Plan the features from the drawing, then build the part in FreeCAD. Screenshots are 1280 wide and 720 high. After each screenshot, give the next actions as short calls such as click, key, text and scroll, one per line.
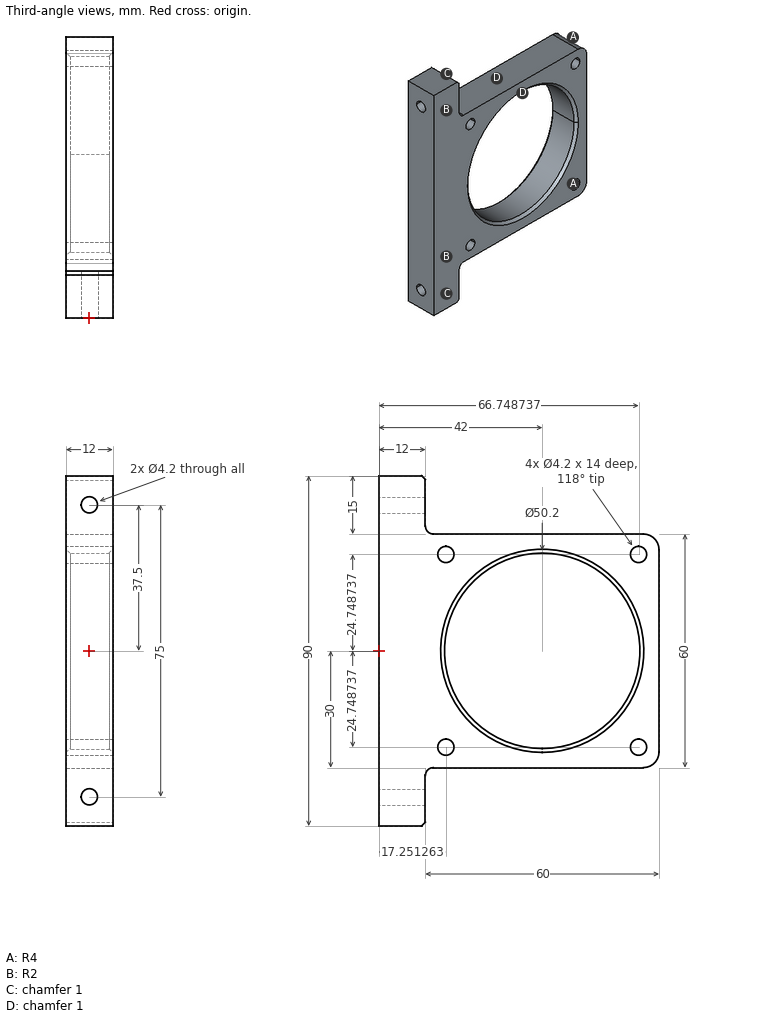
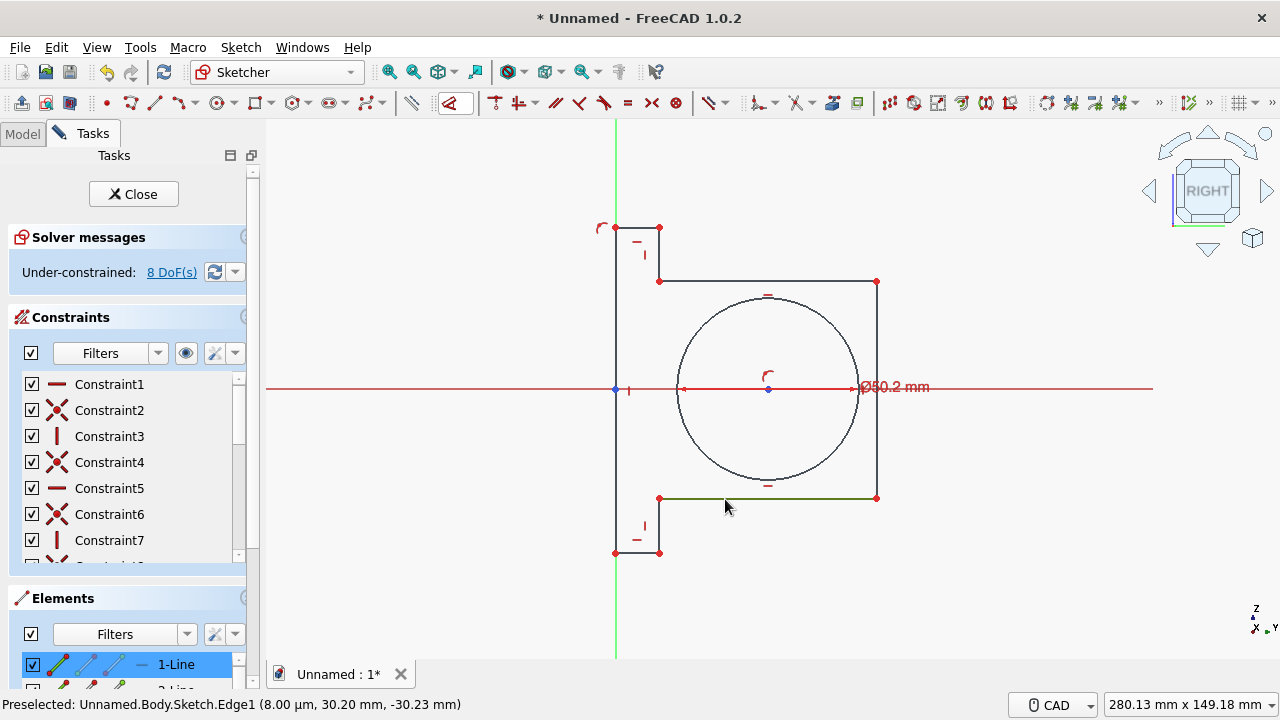
click(468, 104)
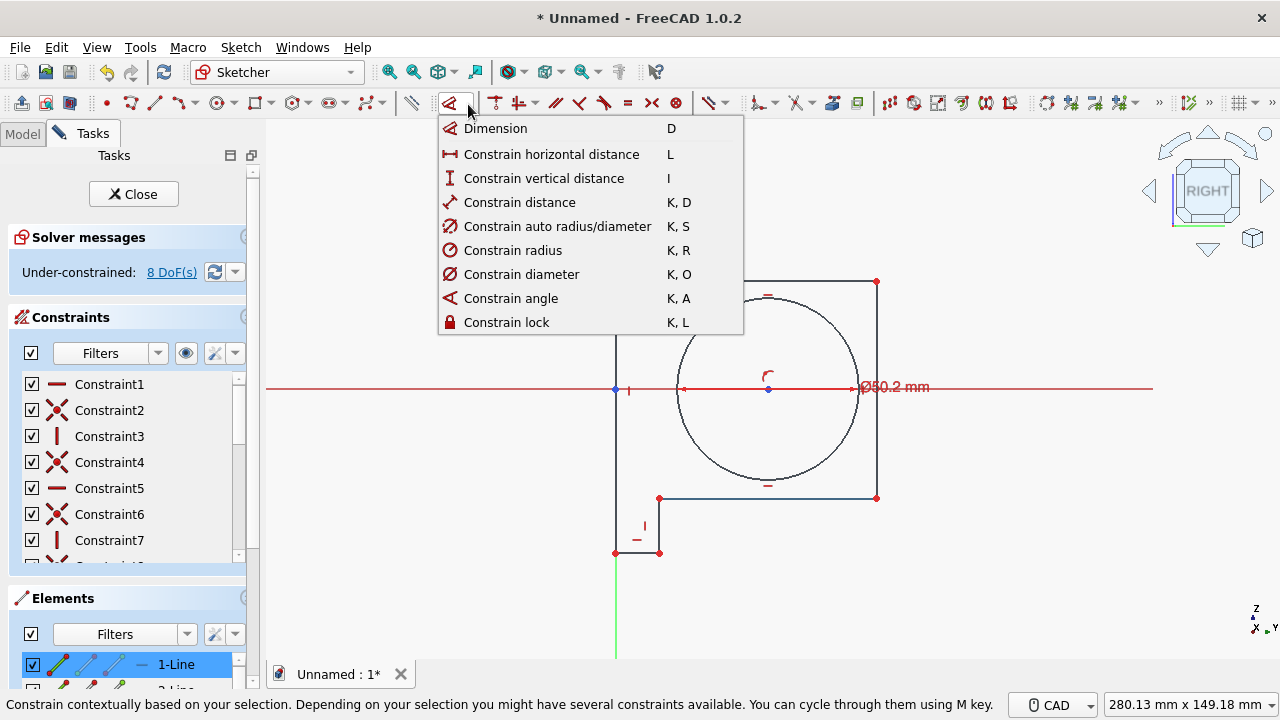
click(591, 154)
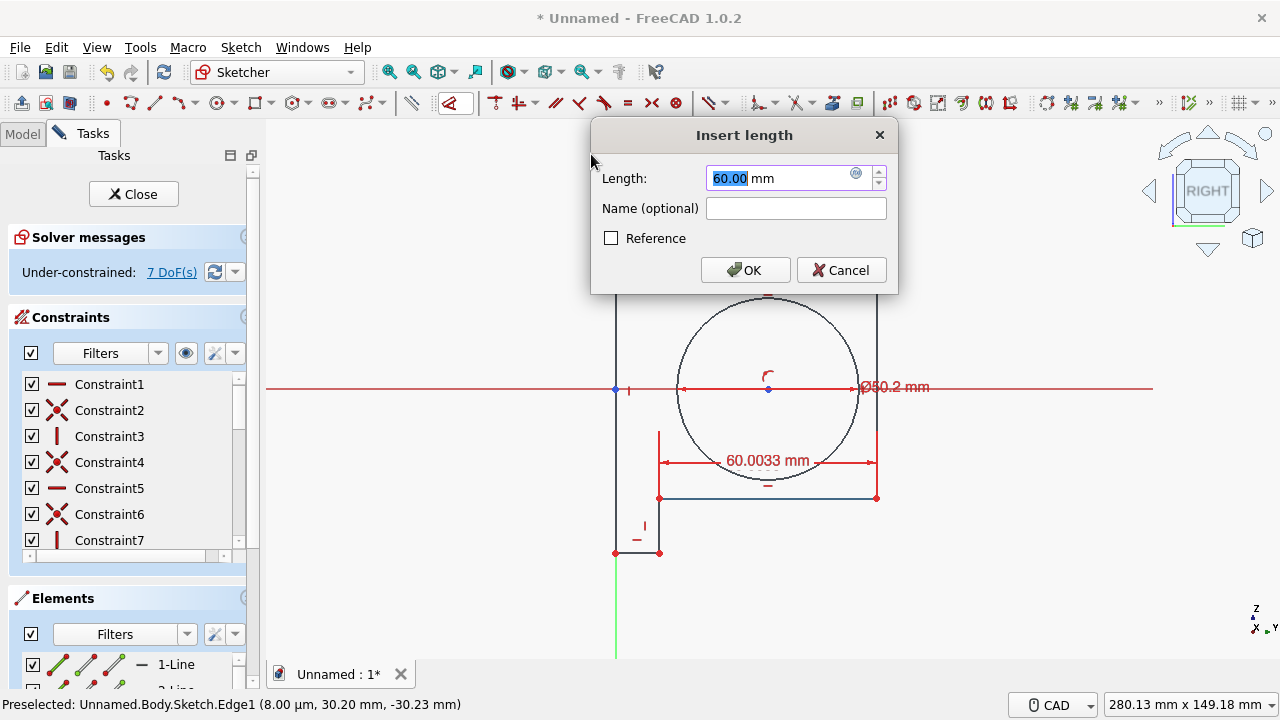
text(60)
key(Return)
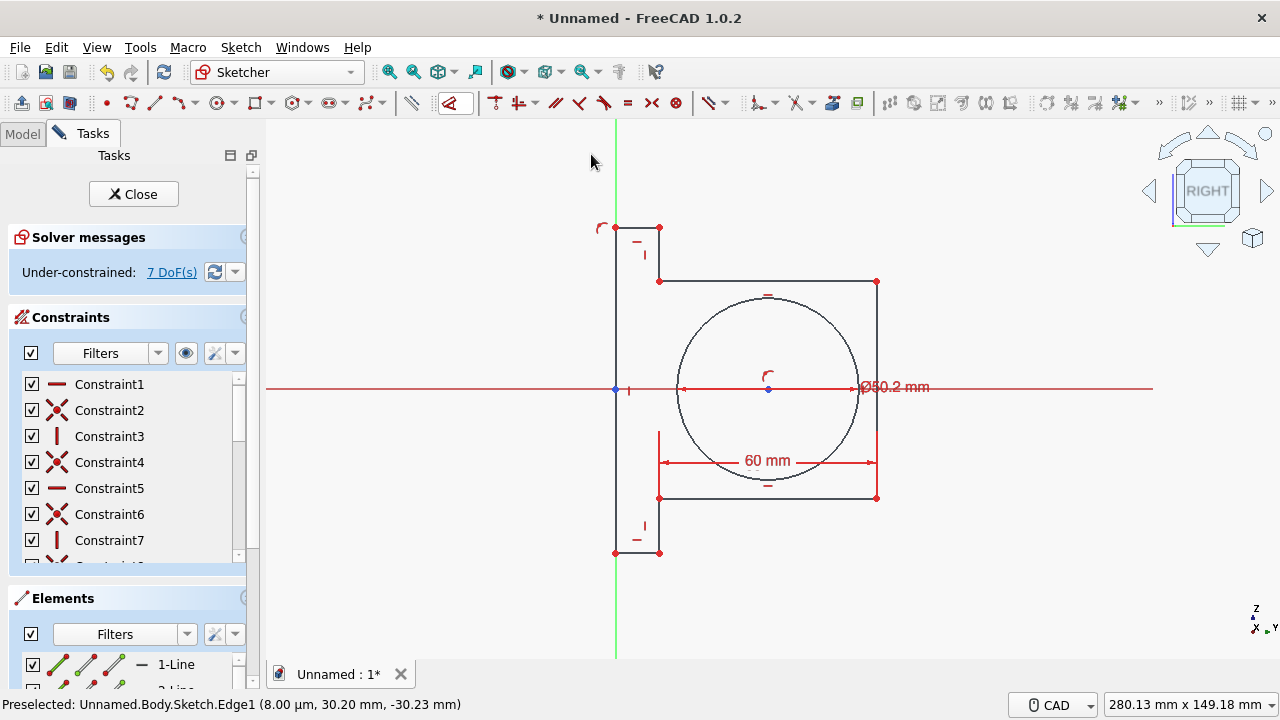
click(877, 433)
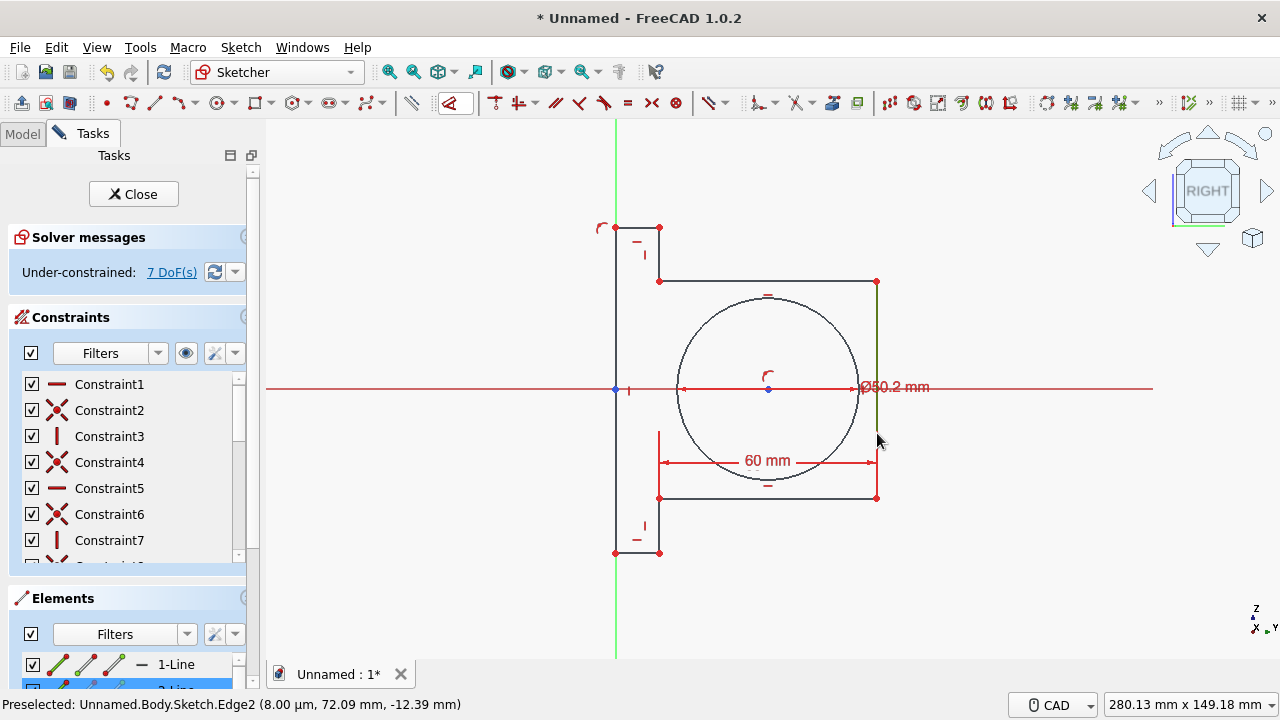
click(468, 104)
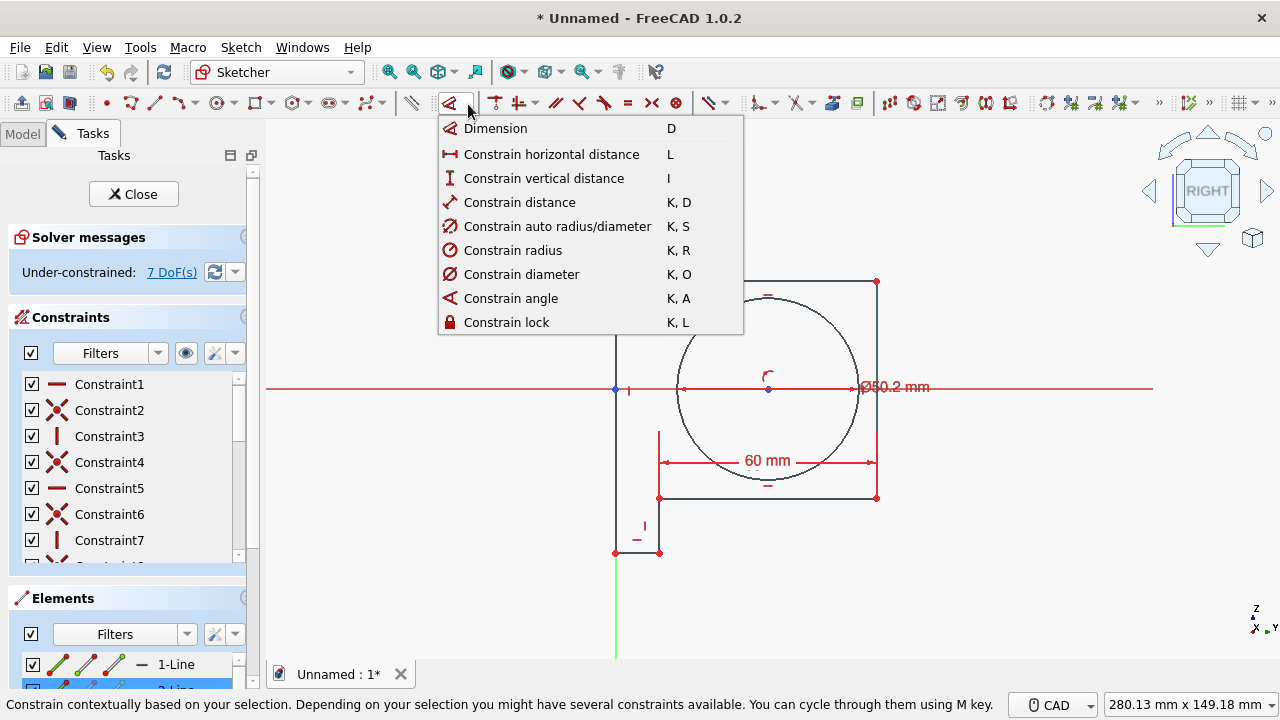
click(591, 178)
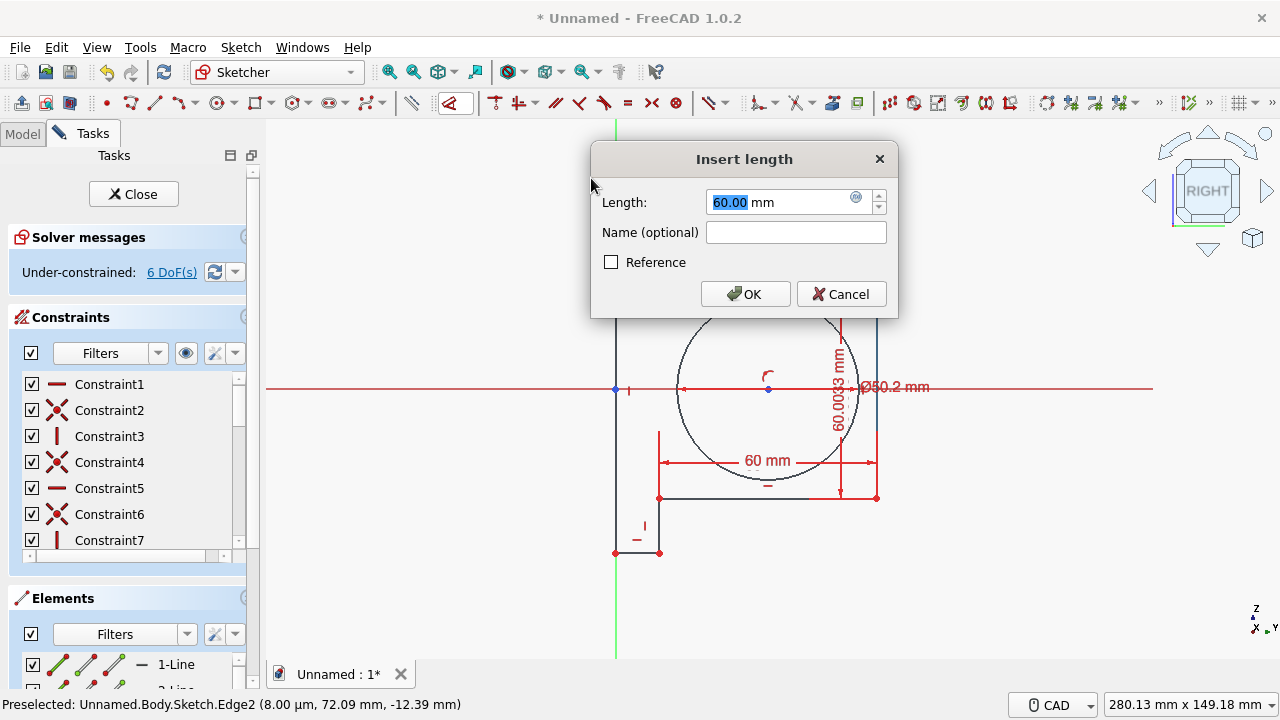
text(60)
key(Return)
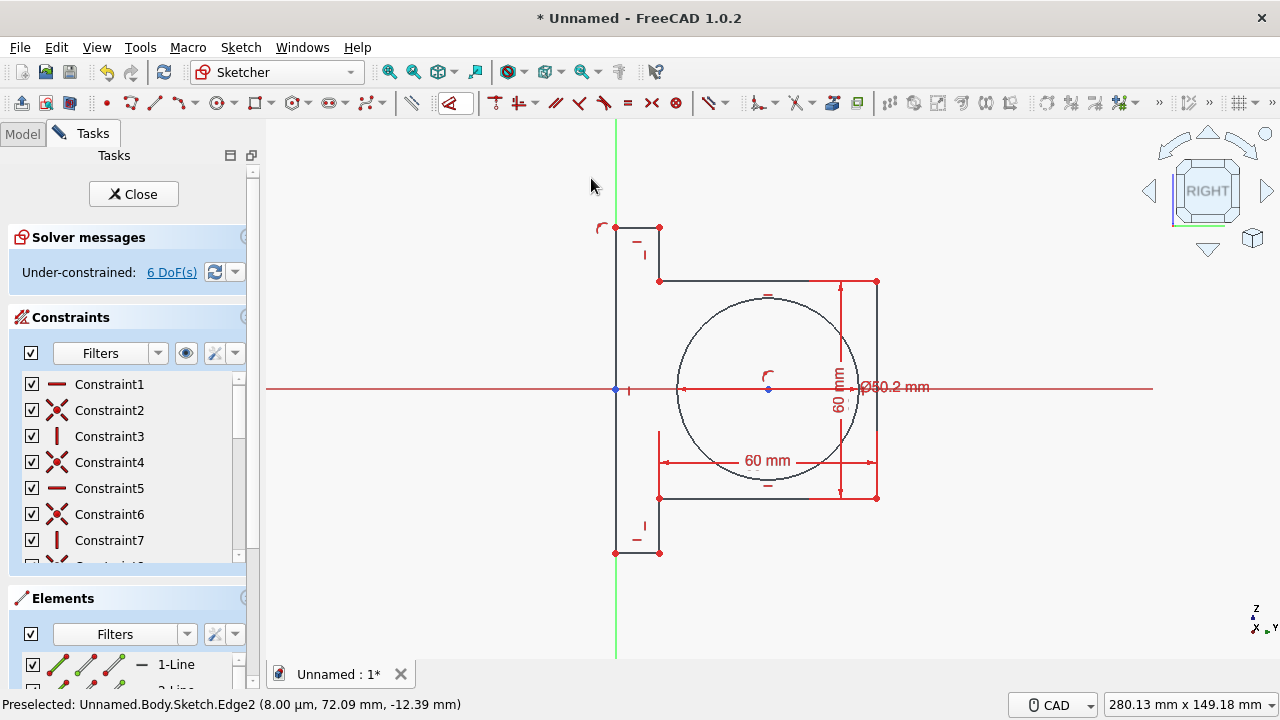
click(811, 281)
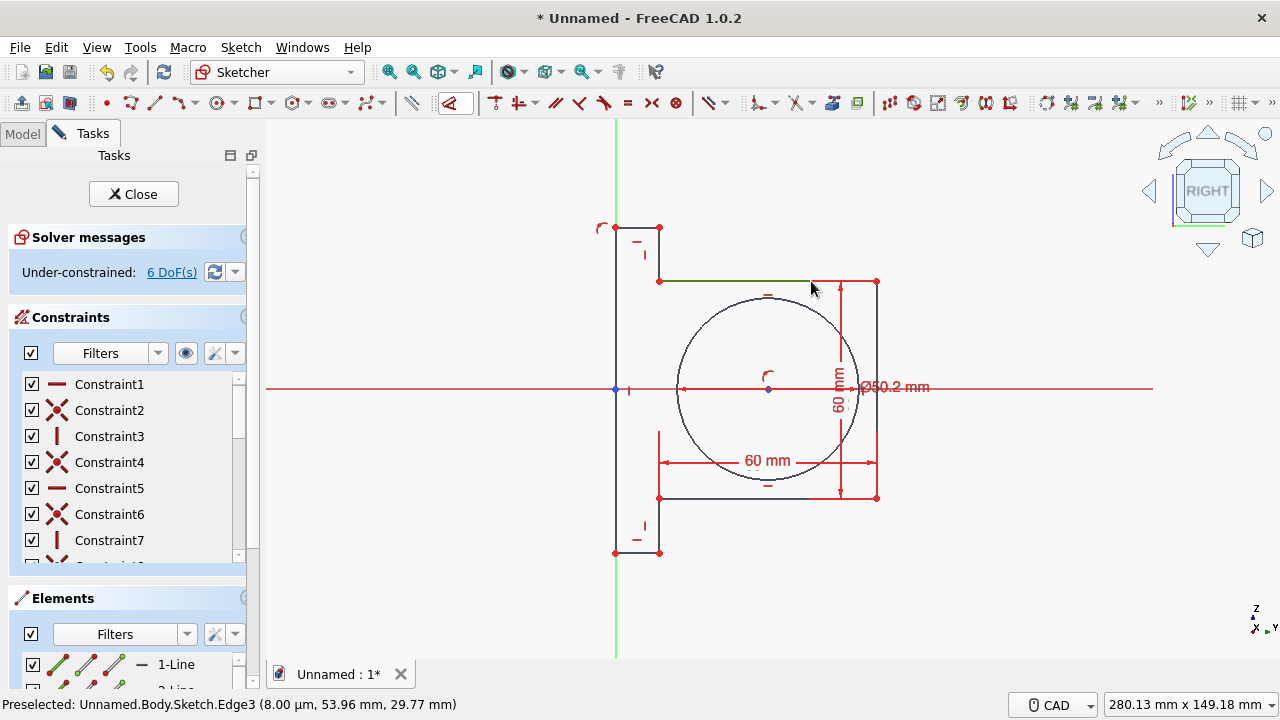
key(l)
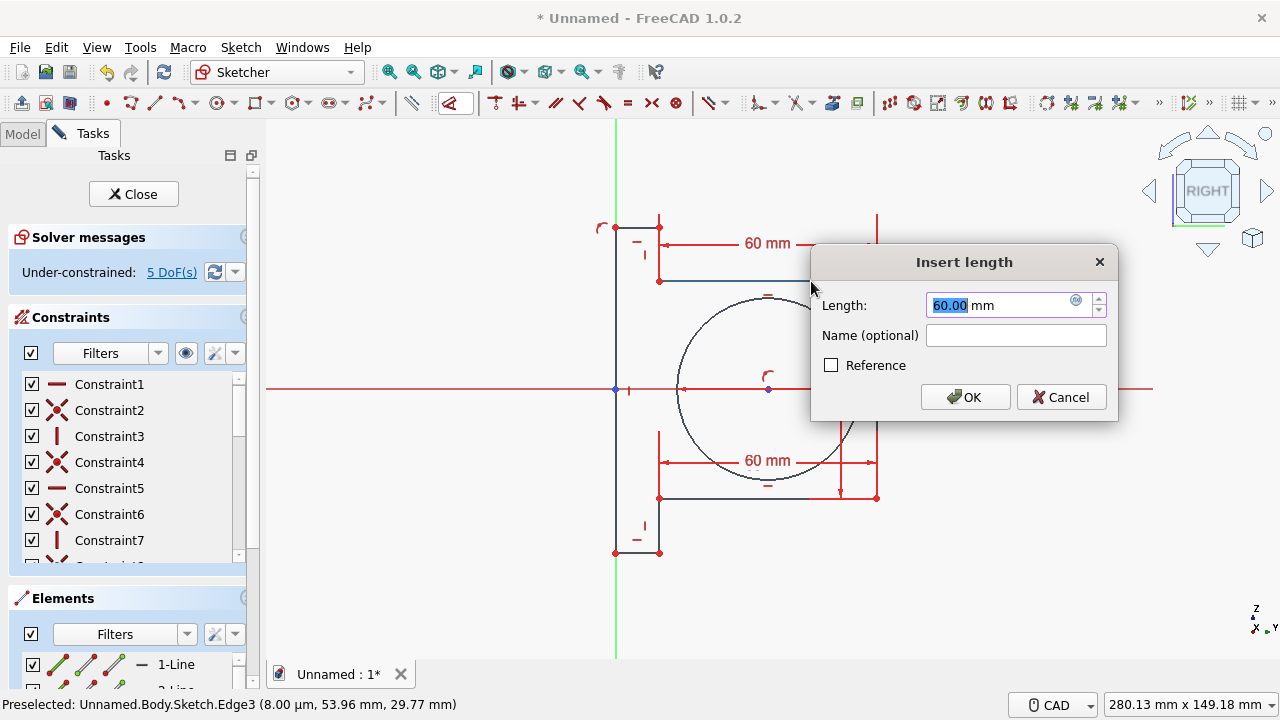
text(60)
key(Return)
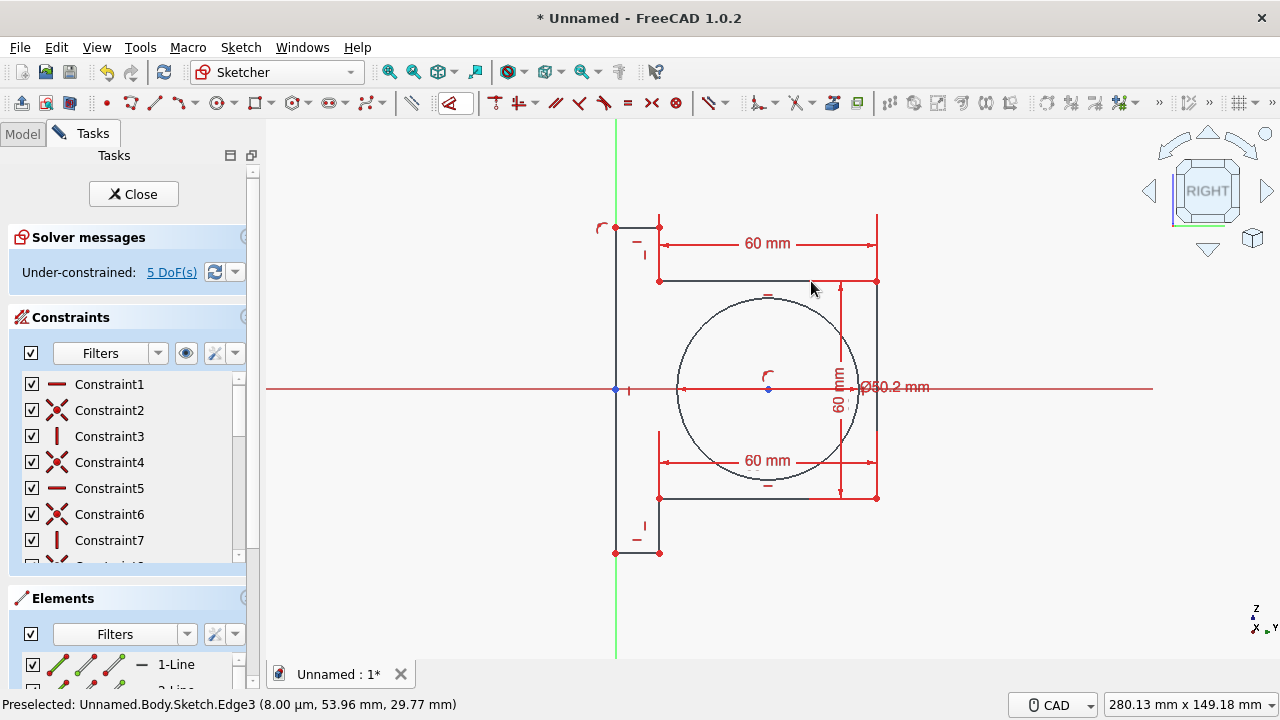
click(659, 265)